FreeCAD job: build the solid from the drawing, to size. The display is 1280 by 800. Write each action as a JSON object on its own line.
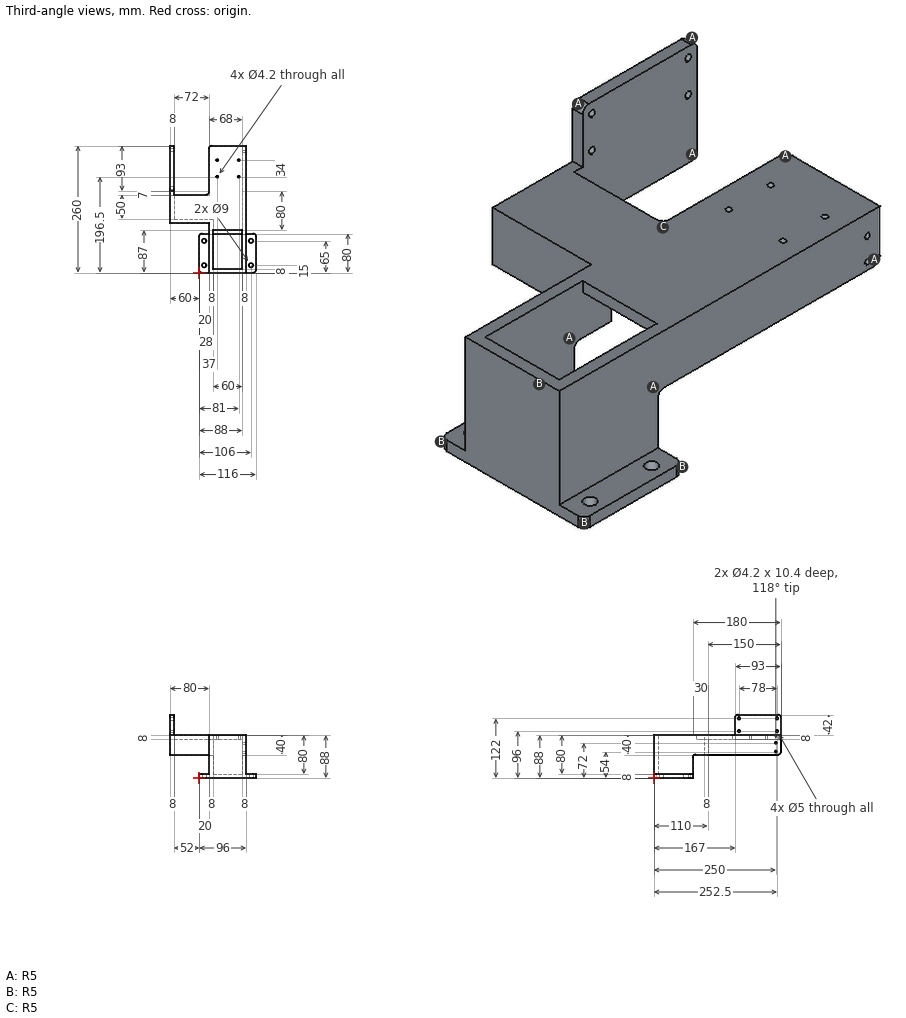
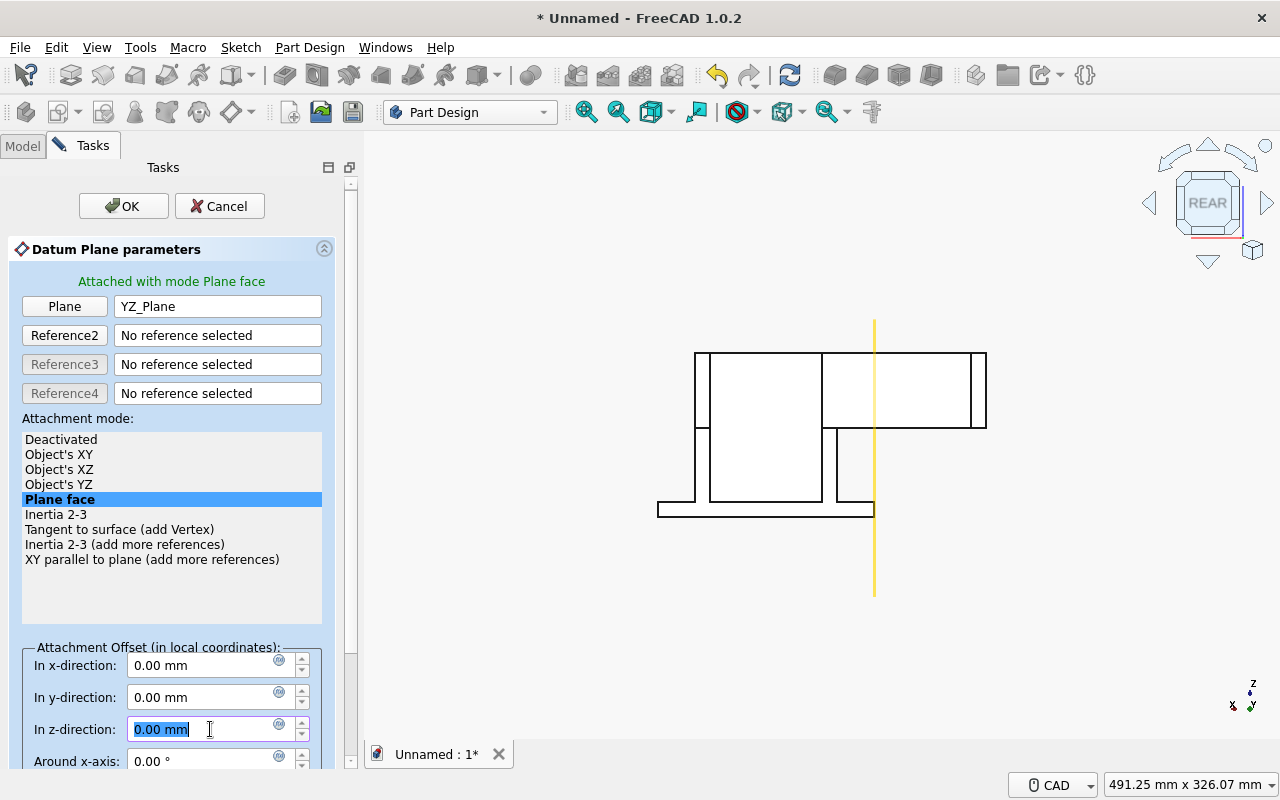
{"action": "type", "text": "88"}
{"action": "key", "text": "Tab"}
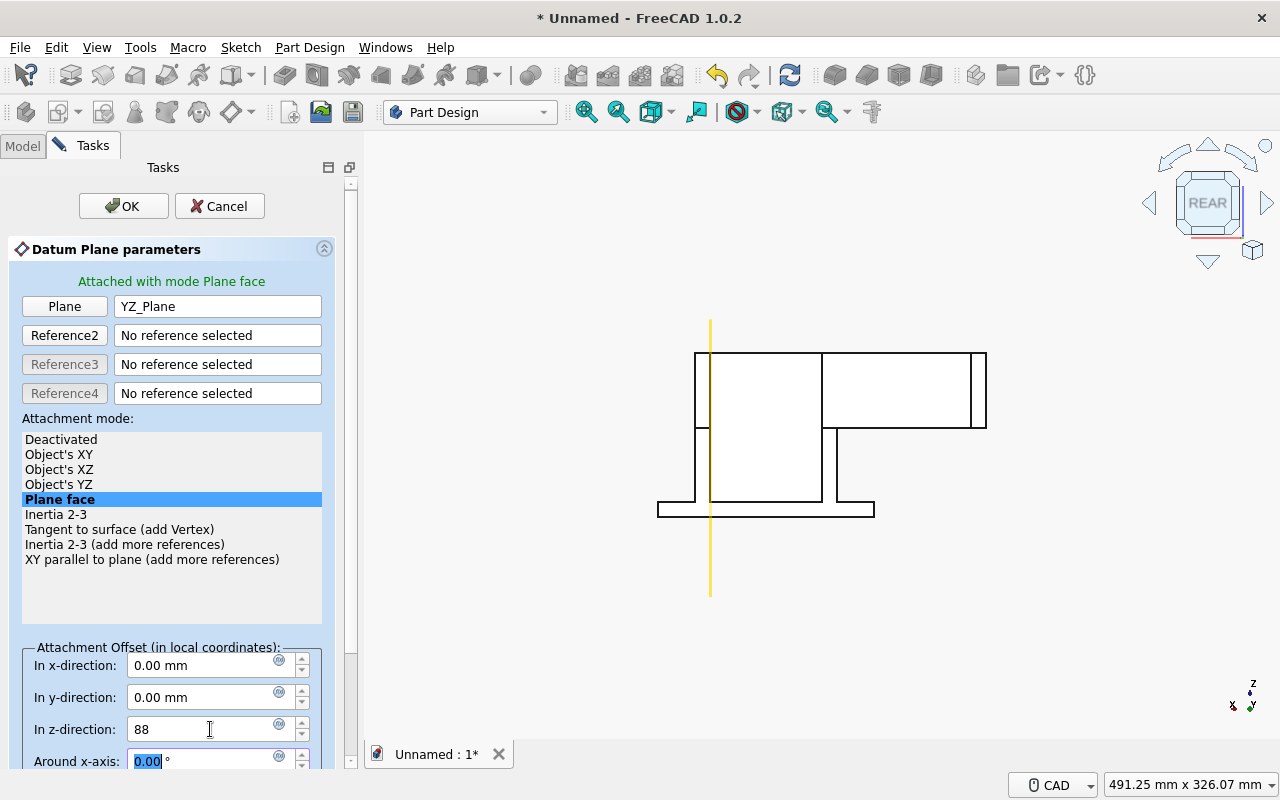
{"action": "left_click", "coordinate": [124, 206]}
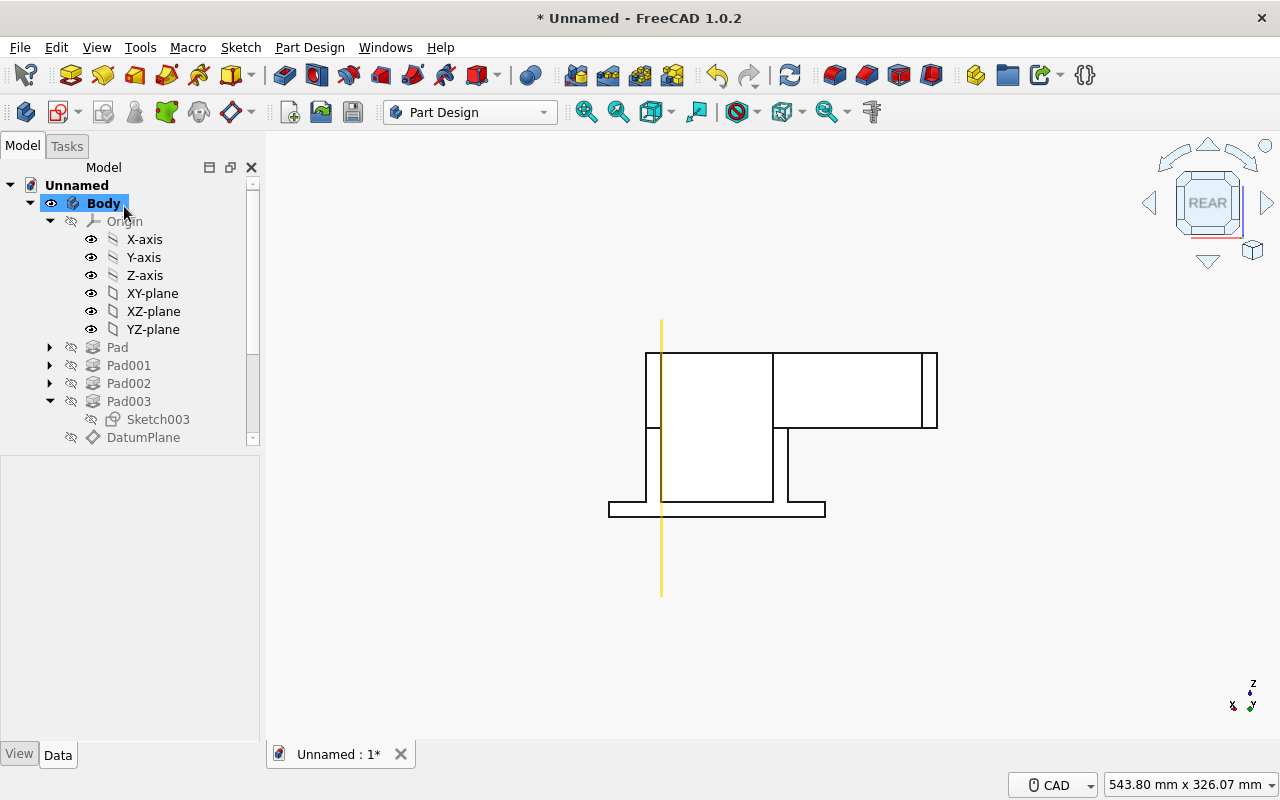
{"action": "scroll", "coordinate": [100, 307], "scroll_direction": "down", "scroll_amount": 3}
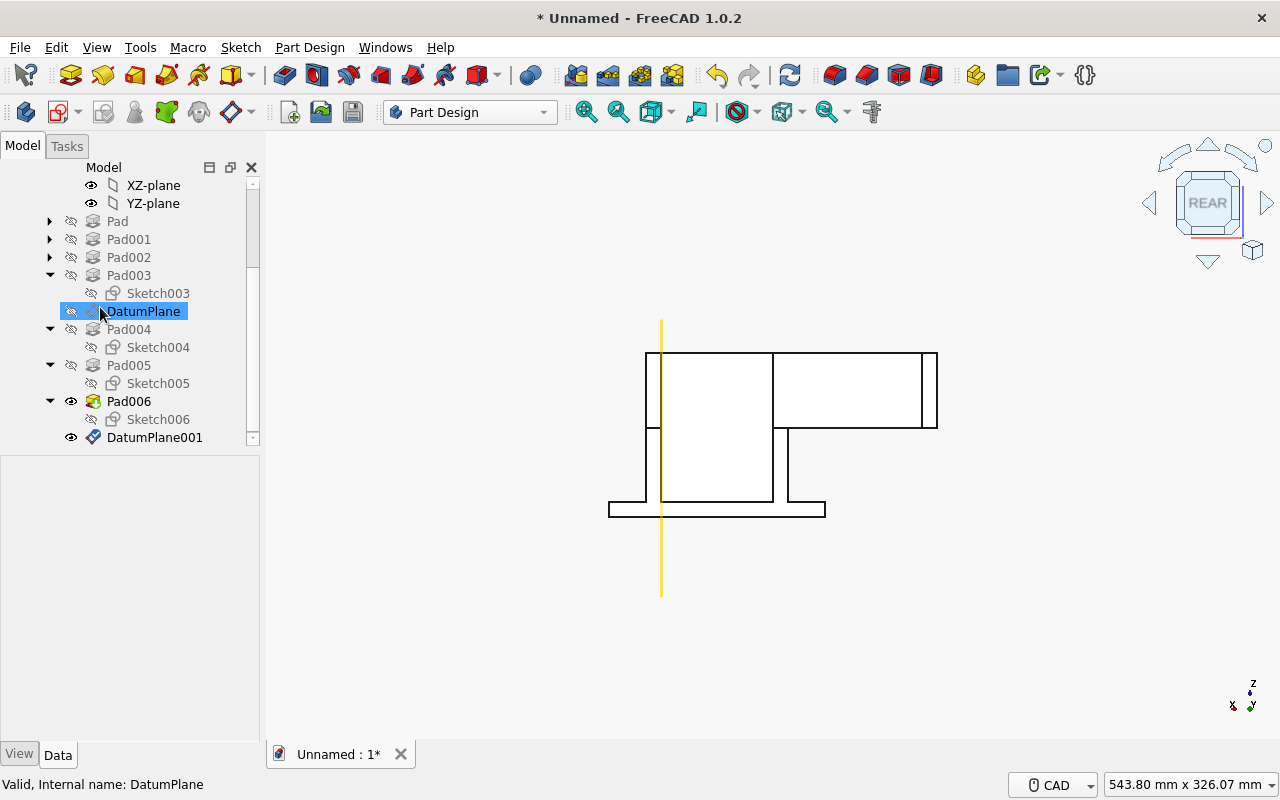
{"action": "left_click", "coordinate": [116, 437]}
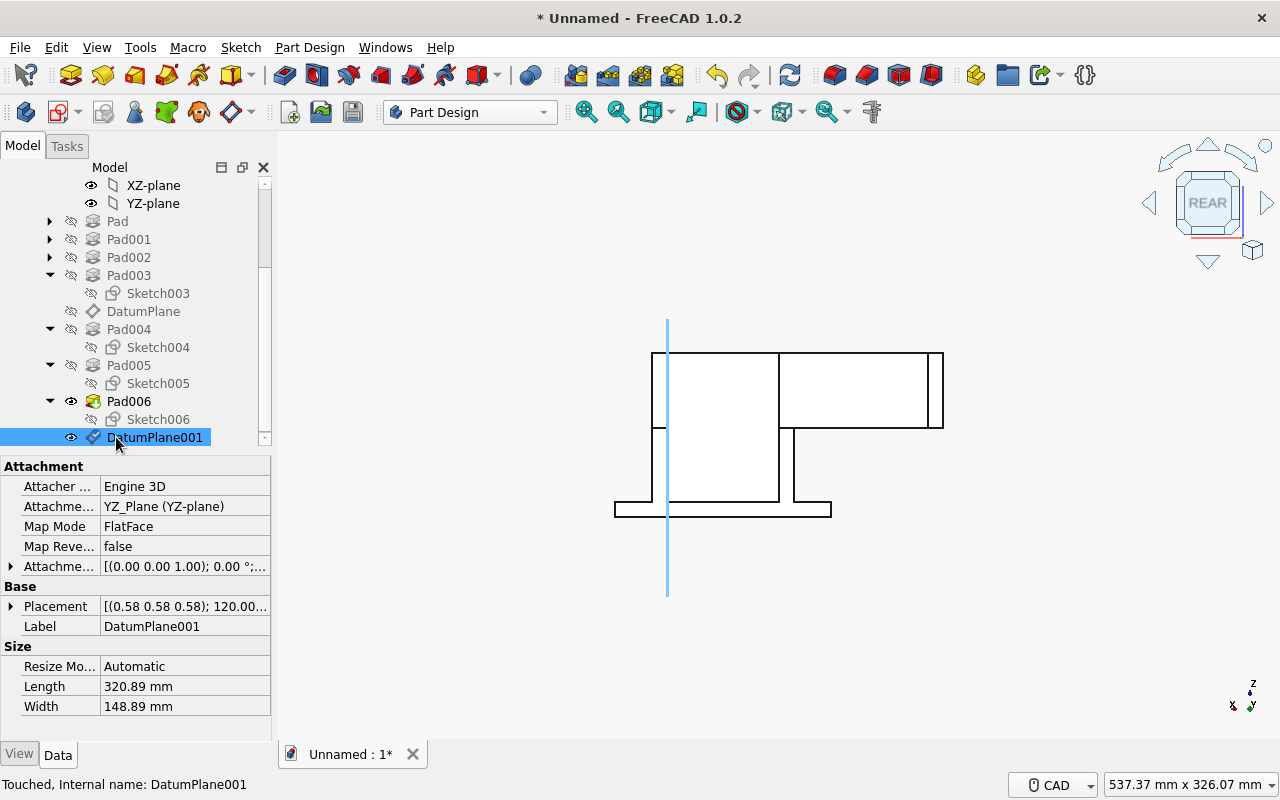
{"action": "left_click", "coordinate": [58, 112]}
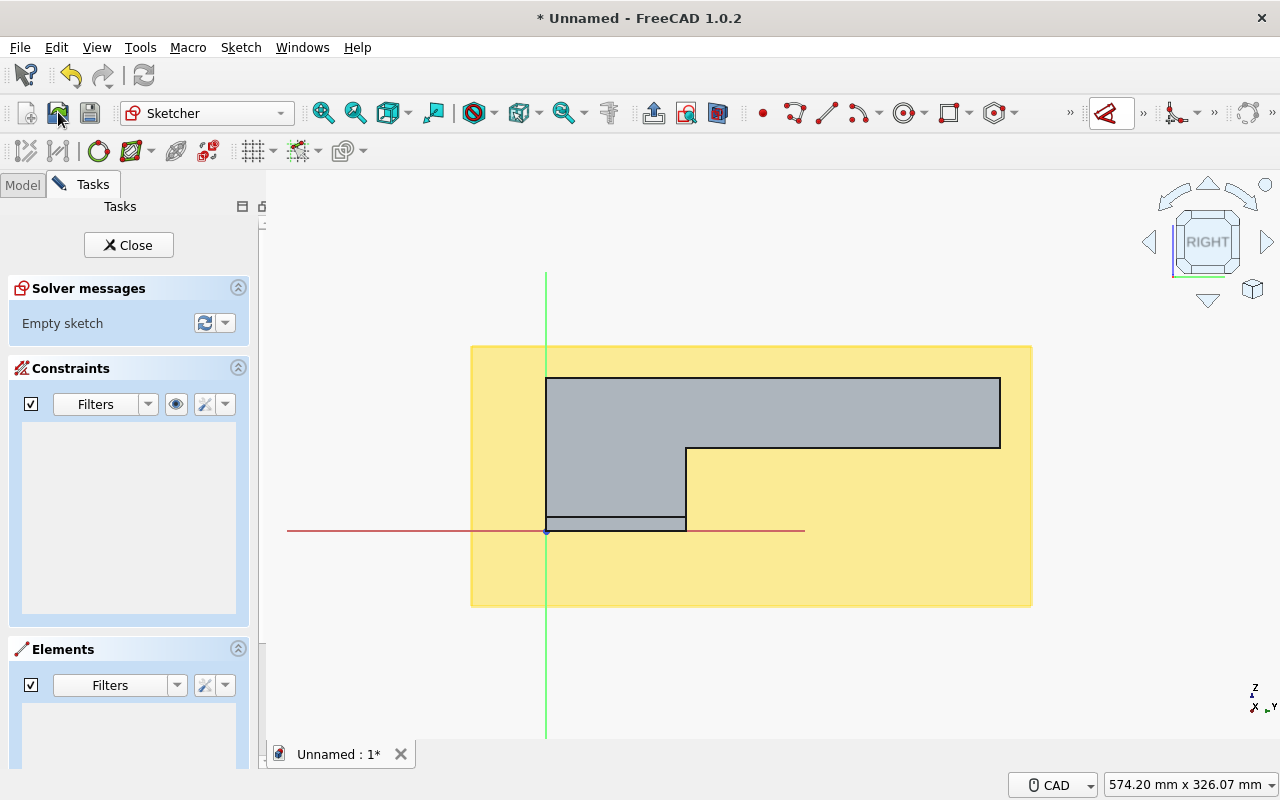
{"action": "left_click", "coordinate": [718, 114]}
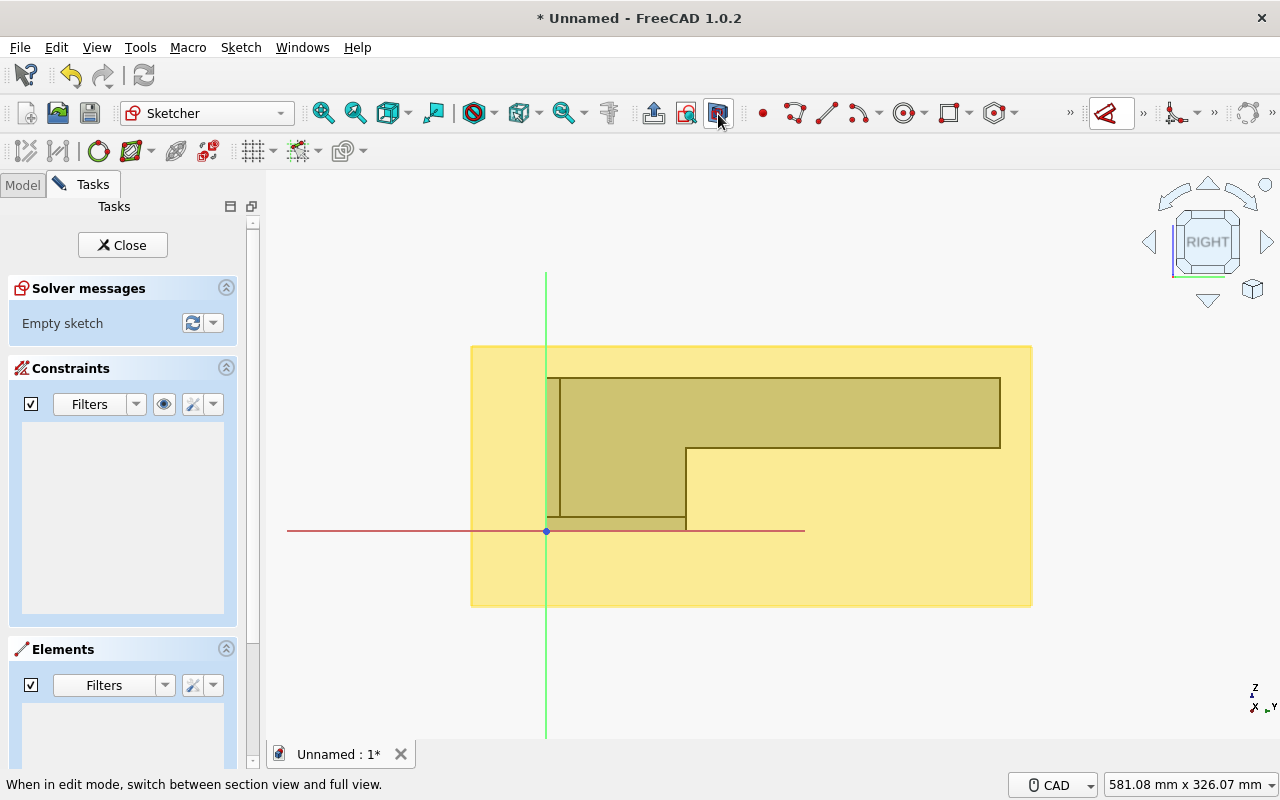
{"action": "scroll", "coordinate": [1011, 355], "scroll_direction": "up", "scroll_amount": 6}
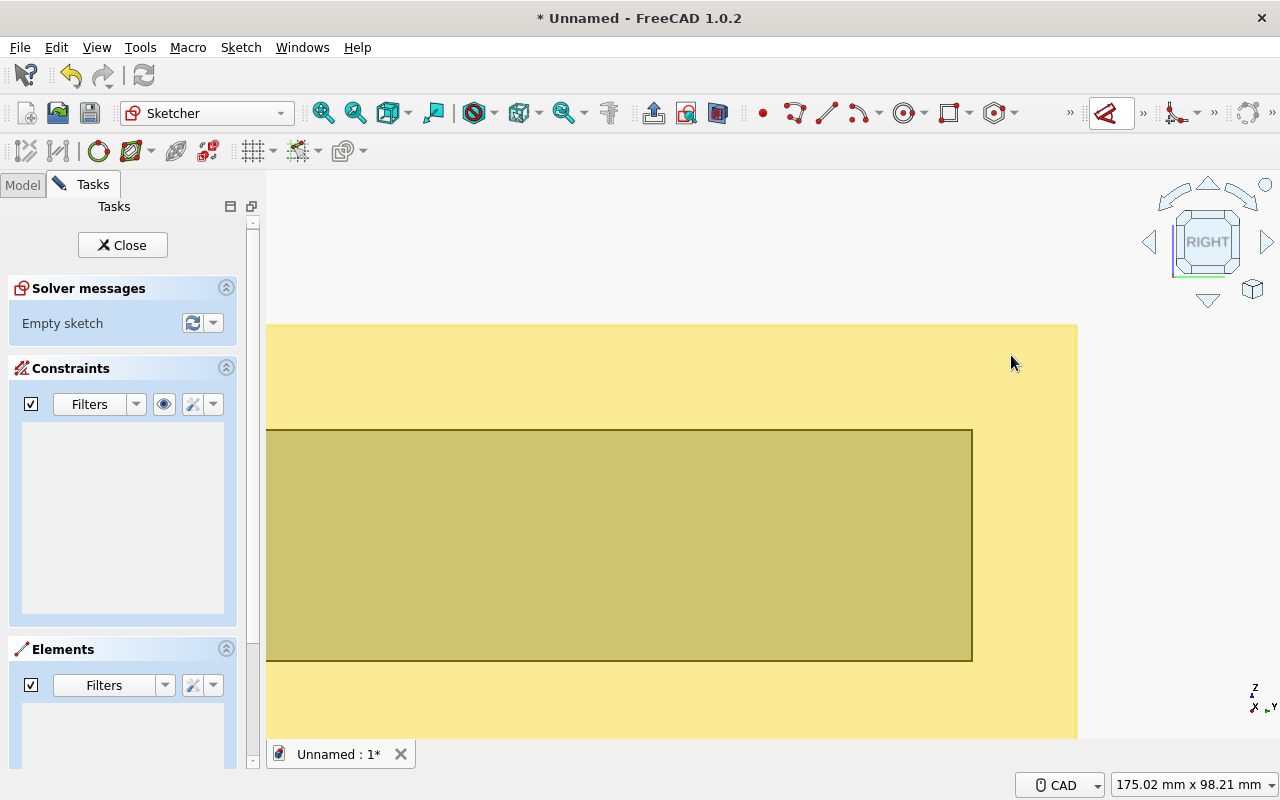
{"action": "left_click", "coordinate": [950, 114]}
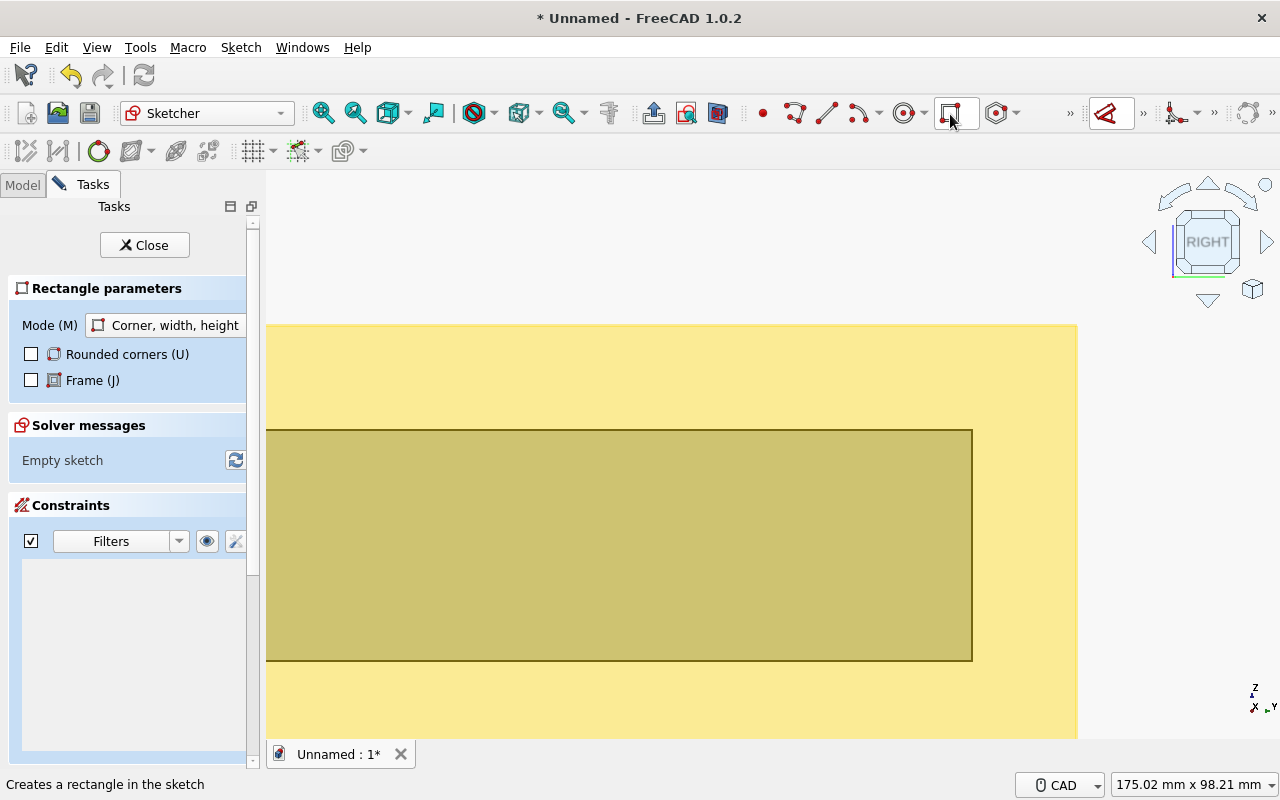
{"action": "left_click", "coordinate": [433, 430]}
{"action": "left_click", "coordinate": [972, 476]}
{"action": "key", "text": "Escape"}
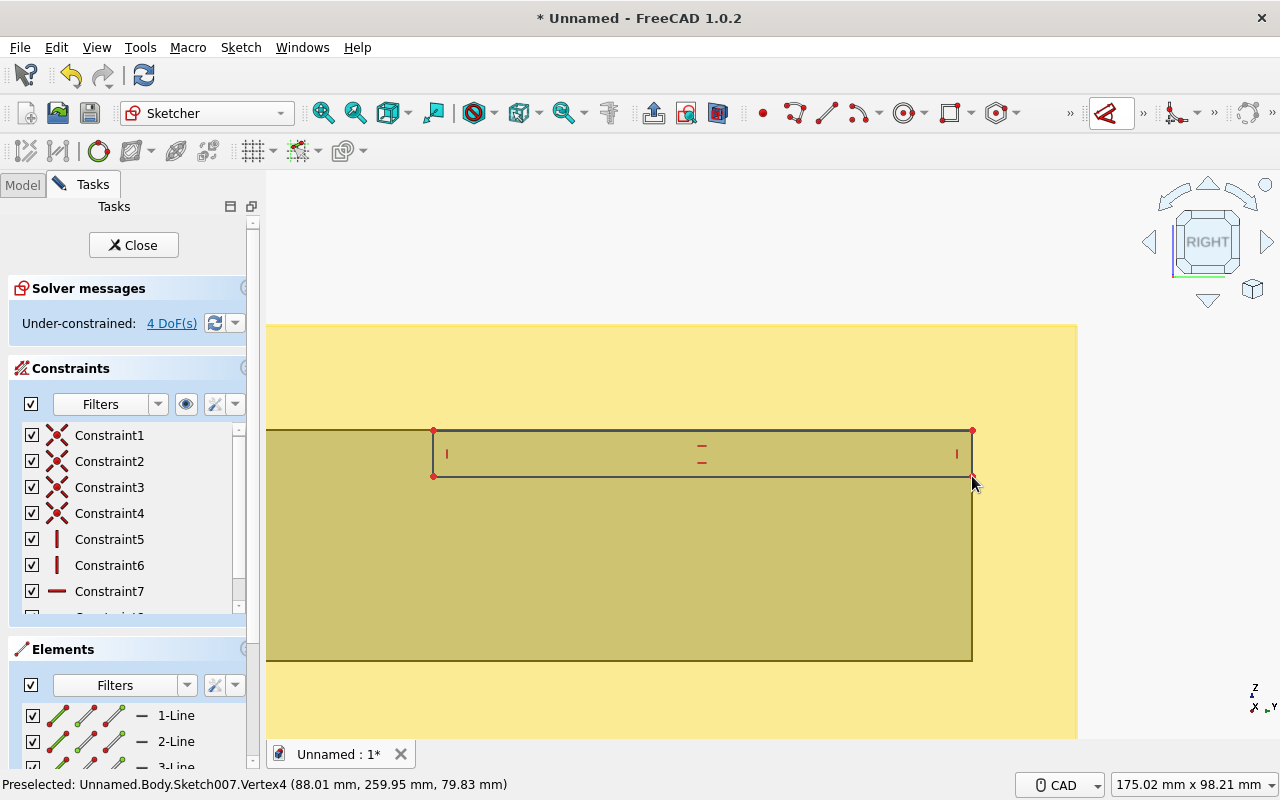
{"action": "left_click", "coordinate": [433, 445]}